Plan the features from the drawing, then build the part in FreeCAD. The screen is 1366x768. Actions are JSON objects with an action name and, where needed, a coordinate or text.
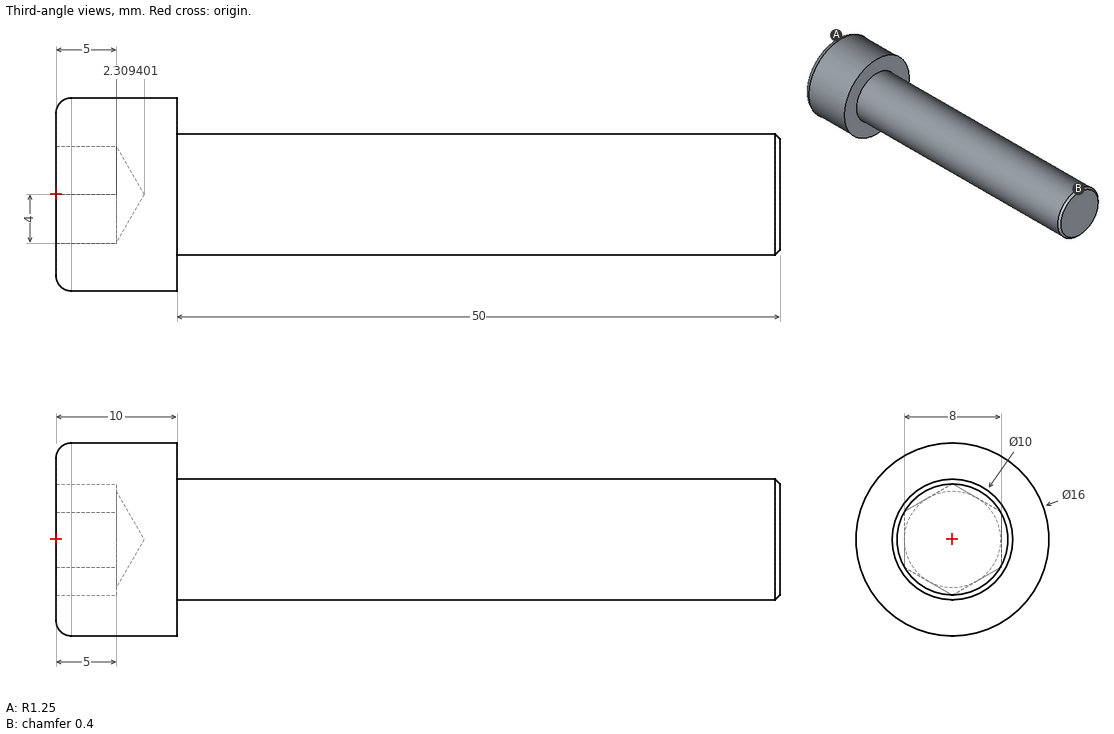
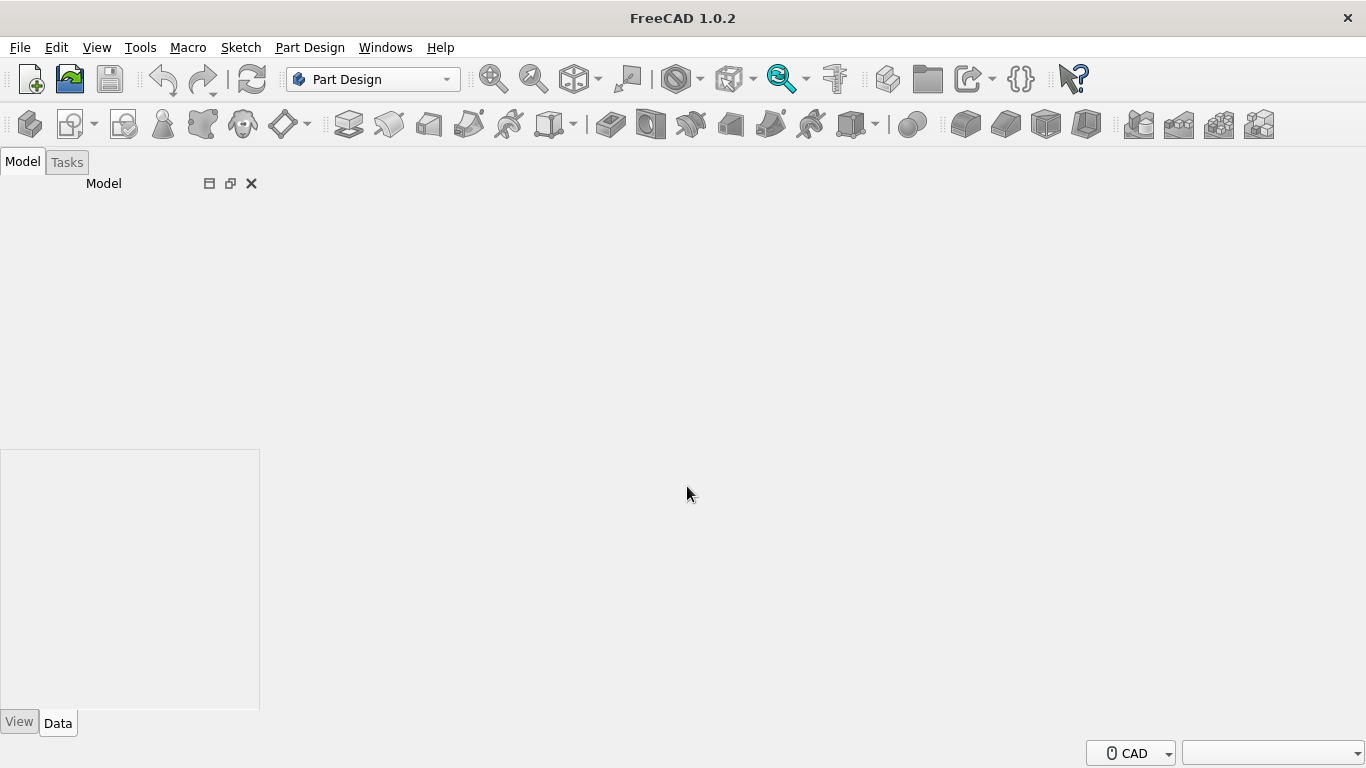
{"action": "left_click", "coordinate": [30, 80]}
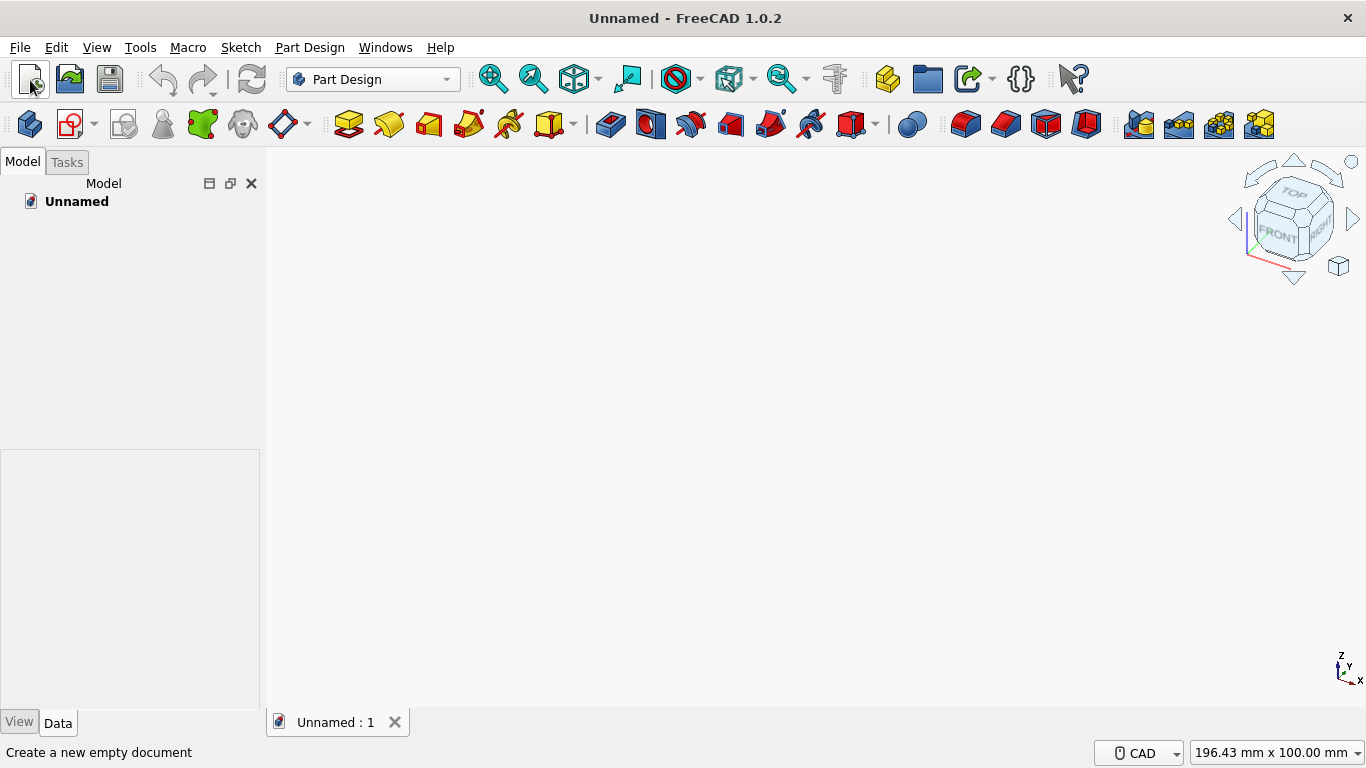
{"action": "left_click", "coordinate": [70, 124]}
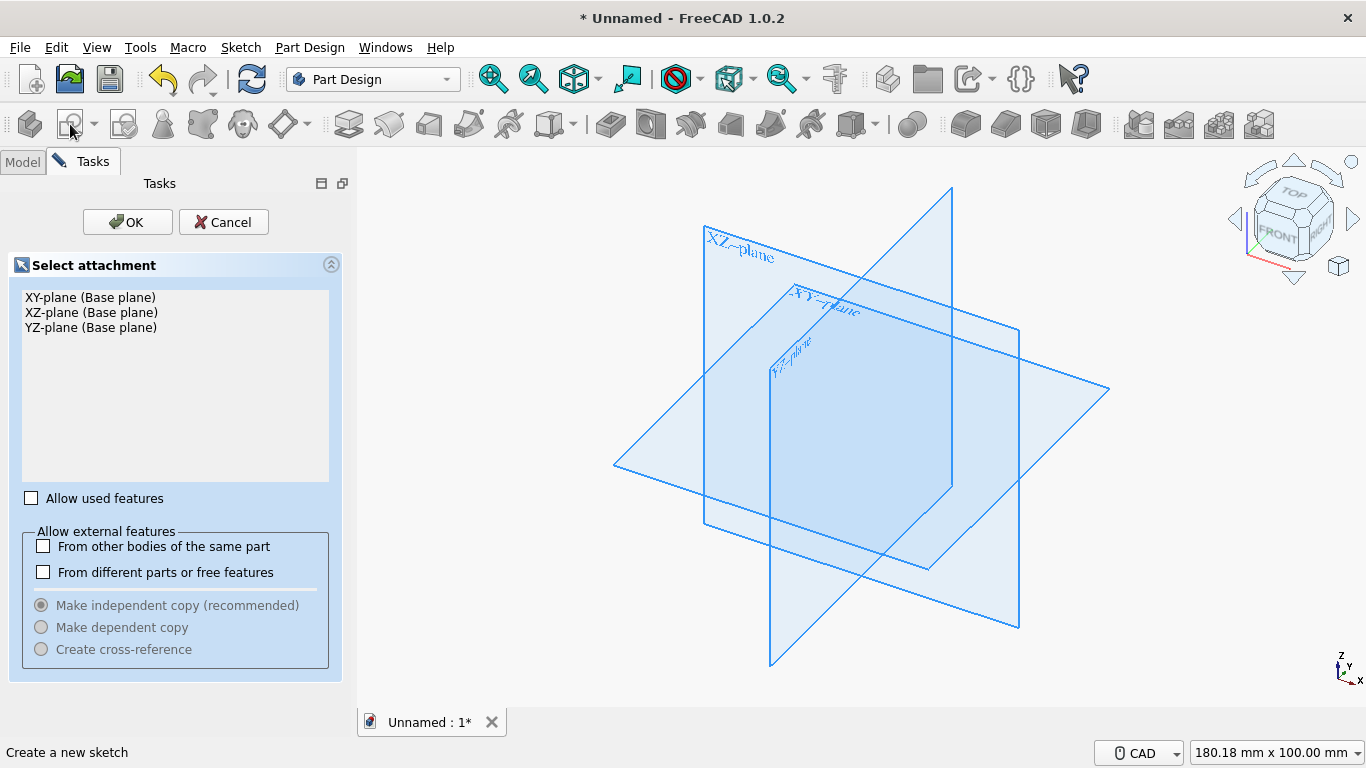
{"action": "left_click", "coordinate": [82, 328]}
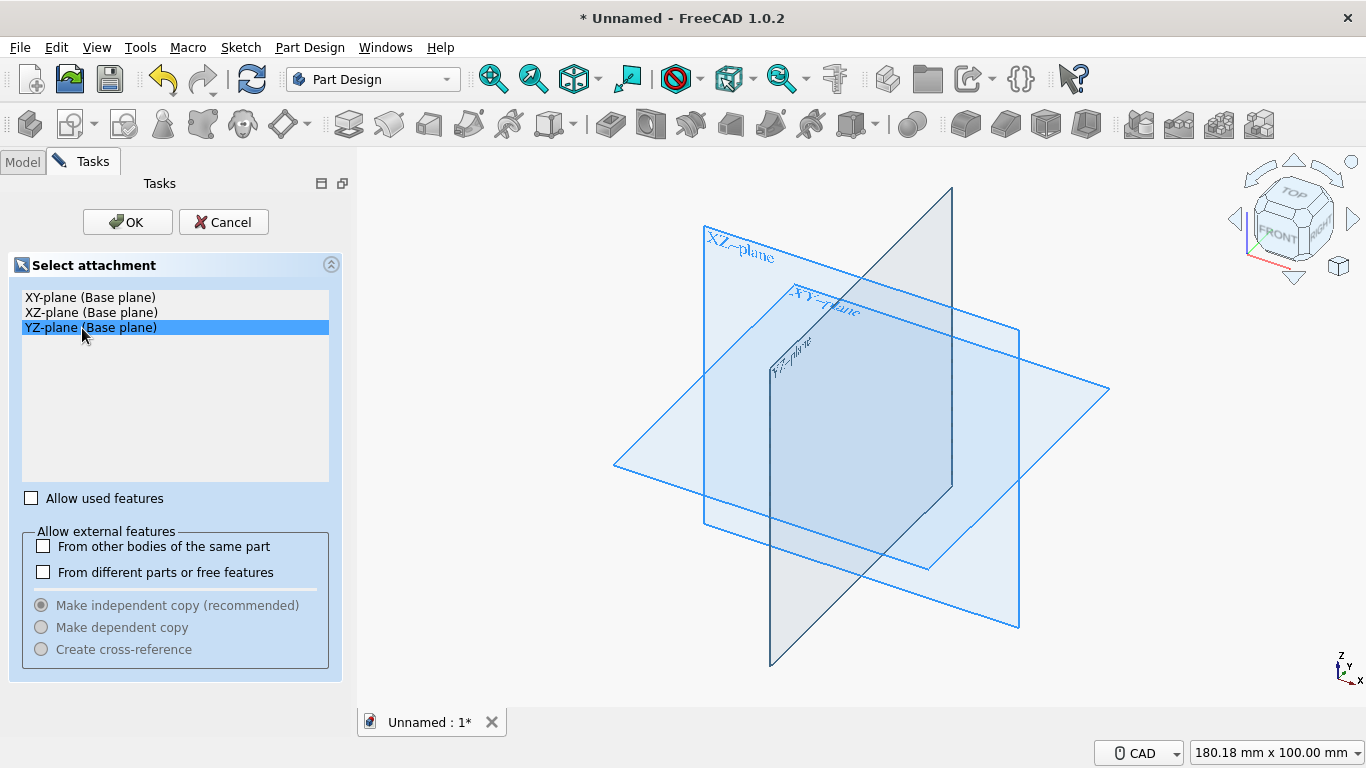
{"action": "left_click", "coordinate": [128, 222]}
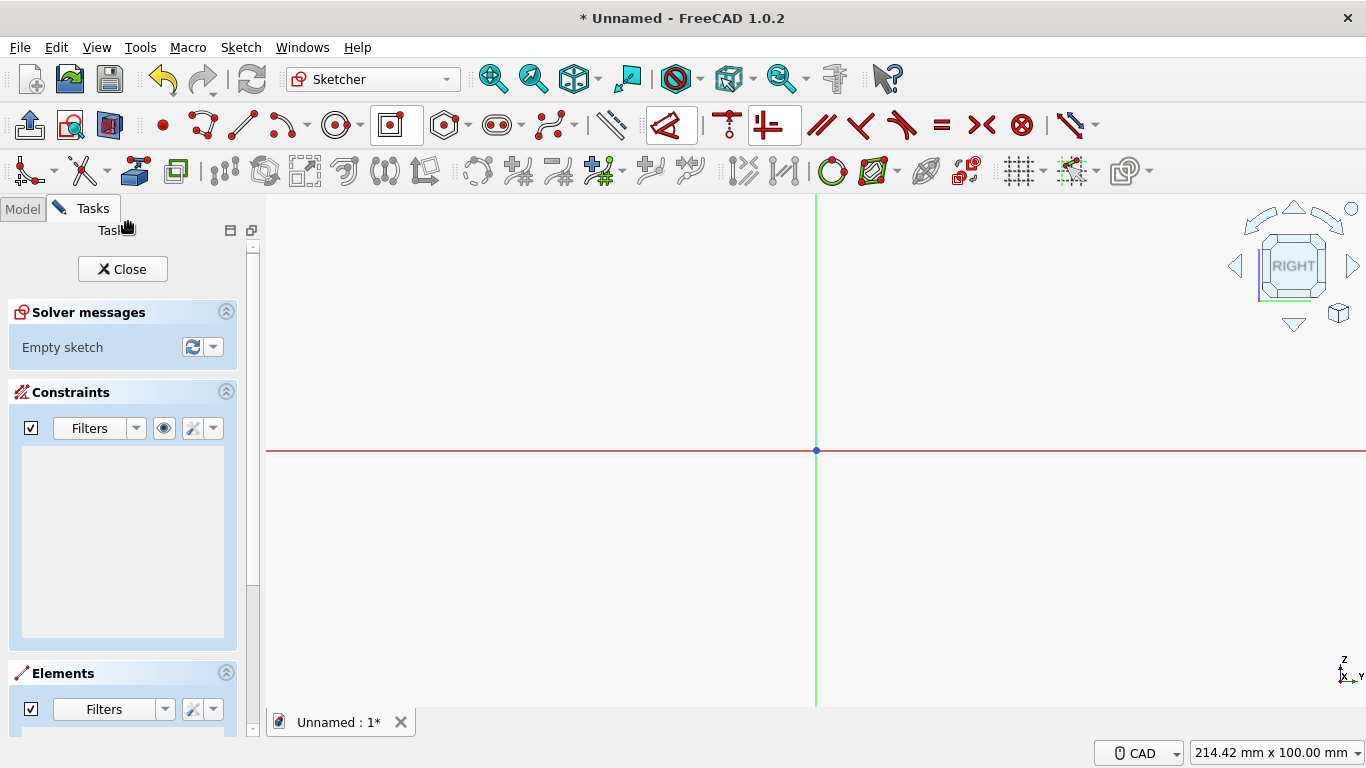
{"action": "scroll", "coordinate": [838, 450], "scroll_direction": "up", "scroll_amount": 7}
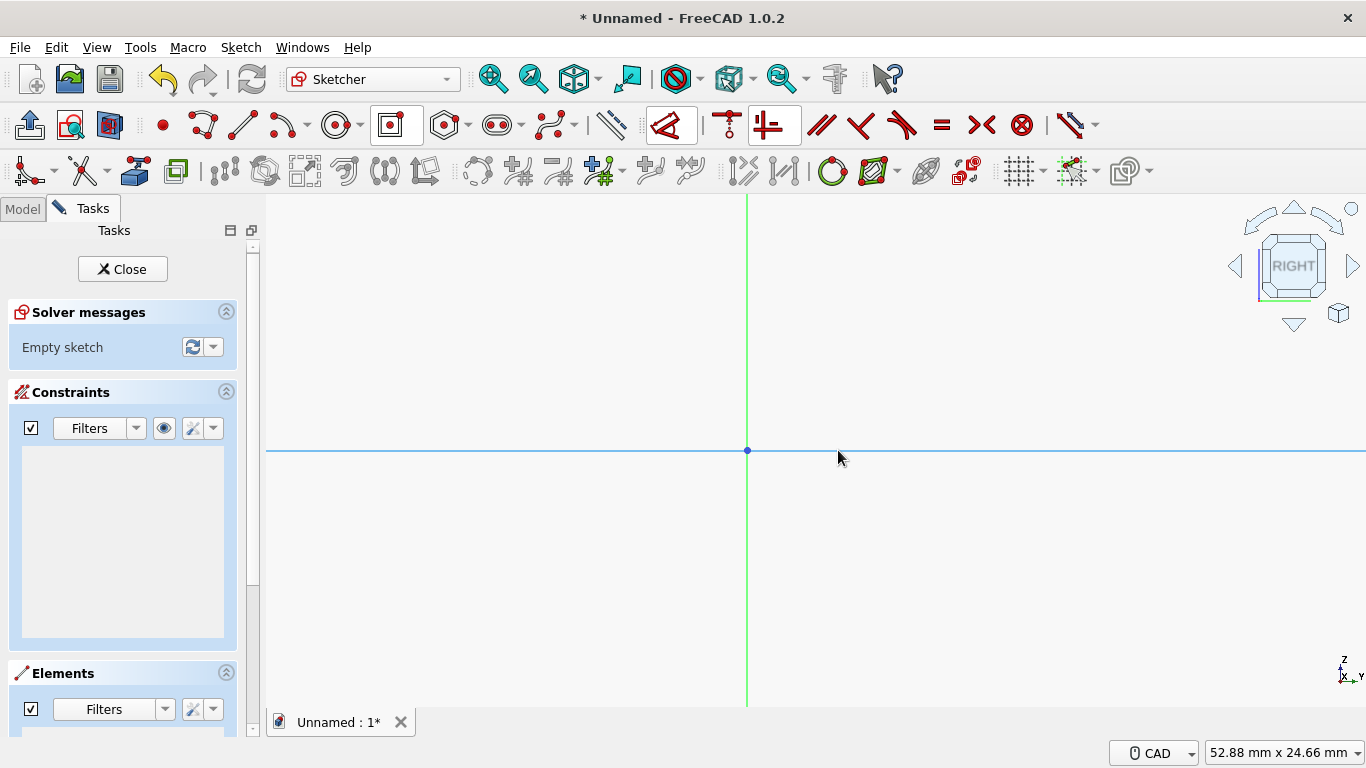
{"action": "left_click", "coordinate": [336, 126]}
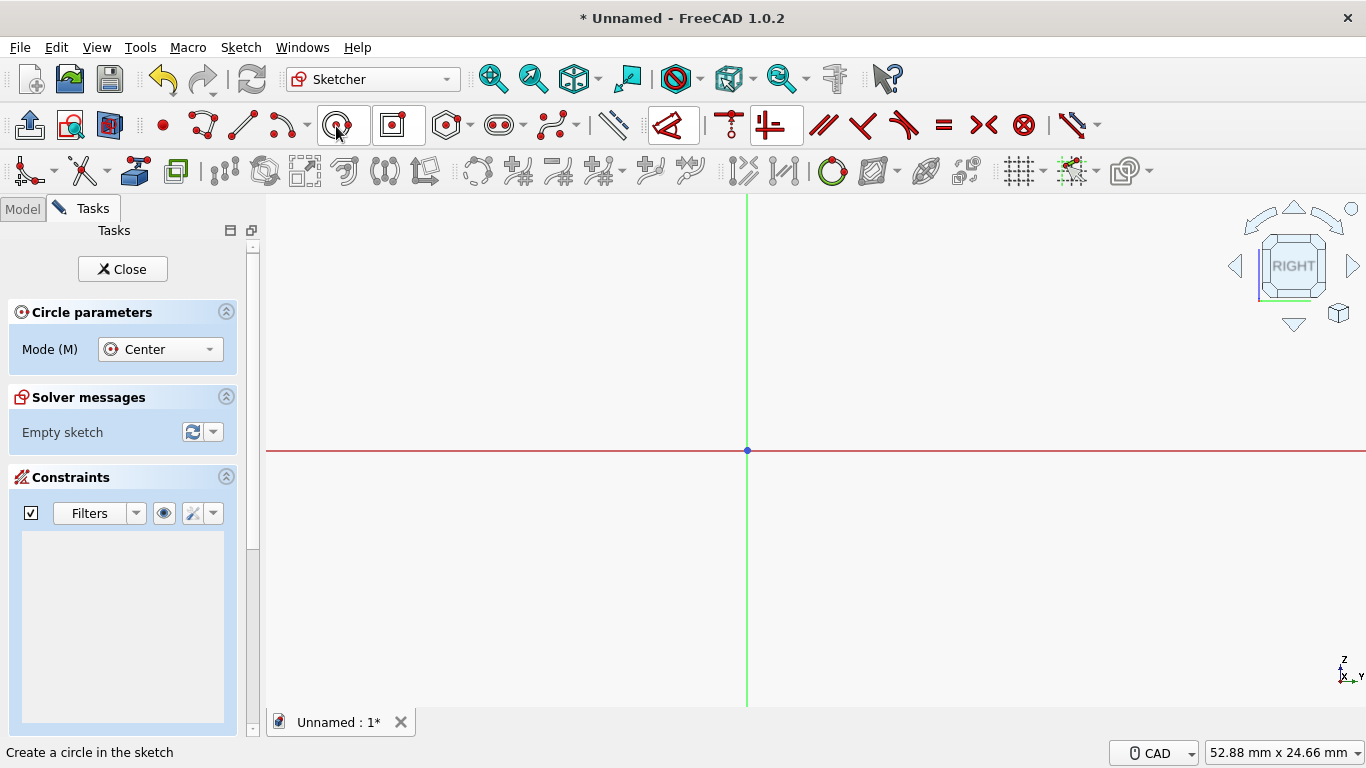
{"action": "left_click", "coordinate": [747, 450]}
{"action": "left_click", "coordinate": [865, 333]}
{"action": "key", "text": "Escape"}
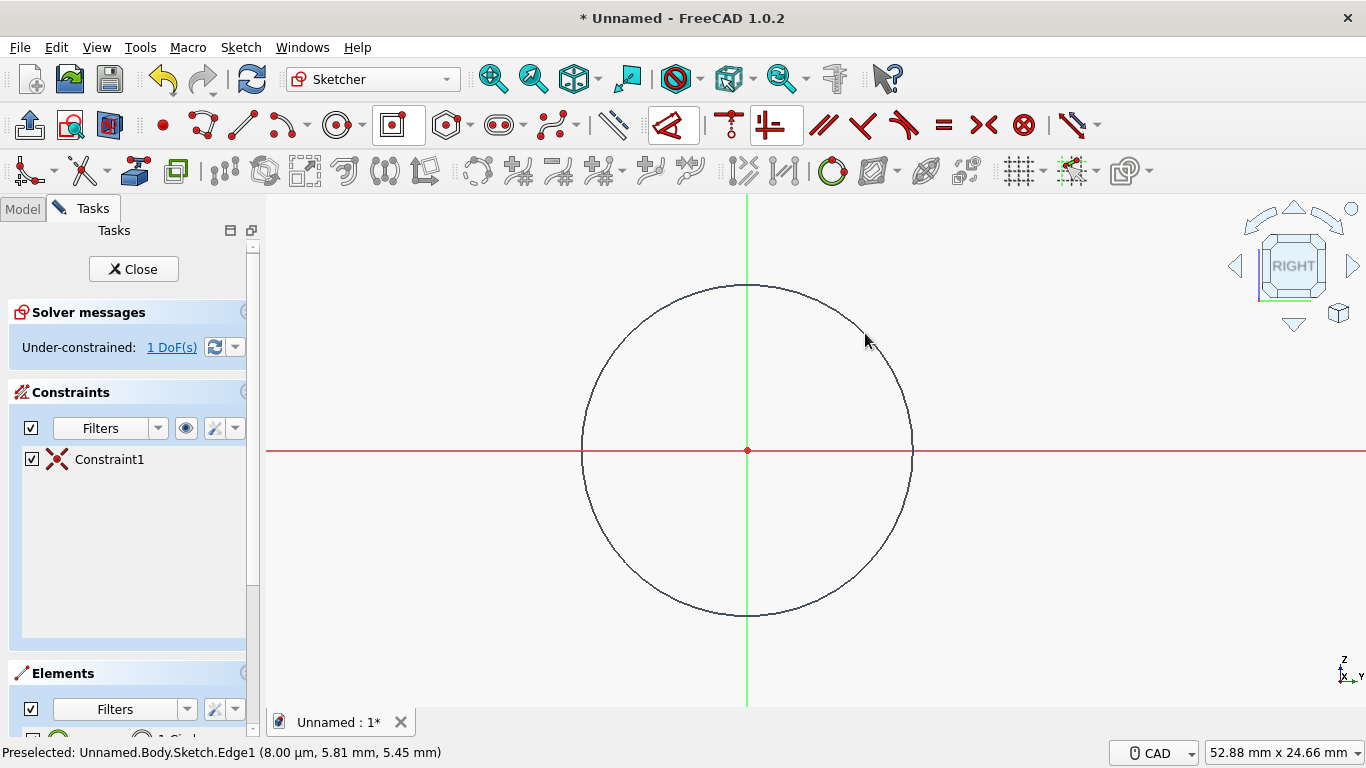
{"action": "left_click", "coordinate": [668, 126]}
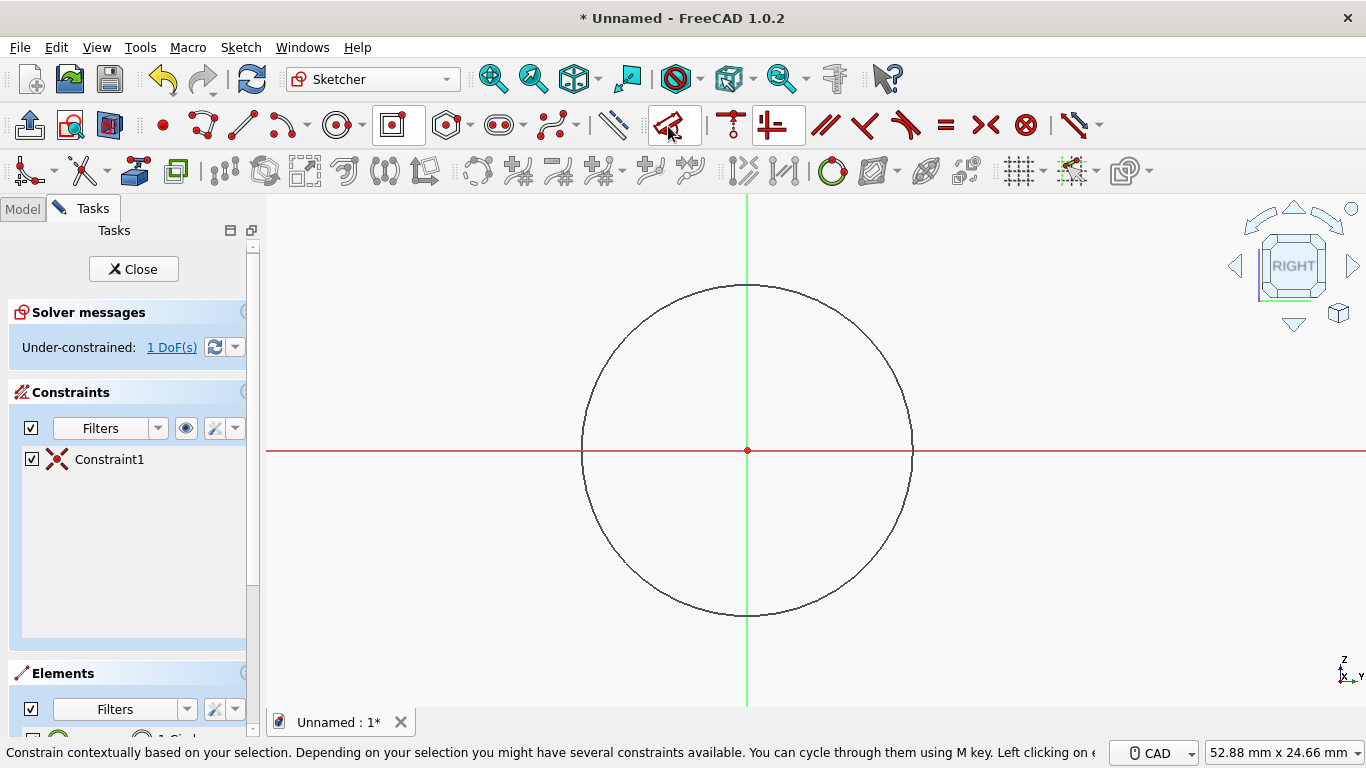
{"action": "left_click", "coordinate": [864, 333]}
{"action": "left_click", "coordinate": [887, 310]}